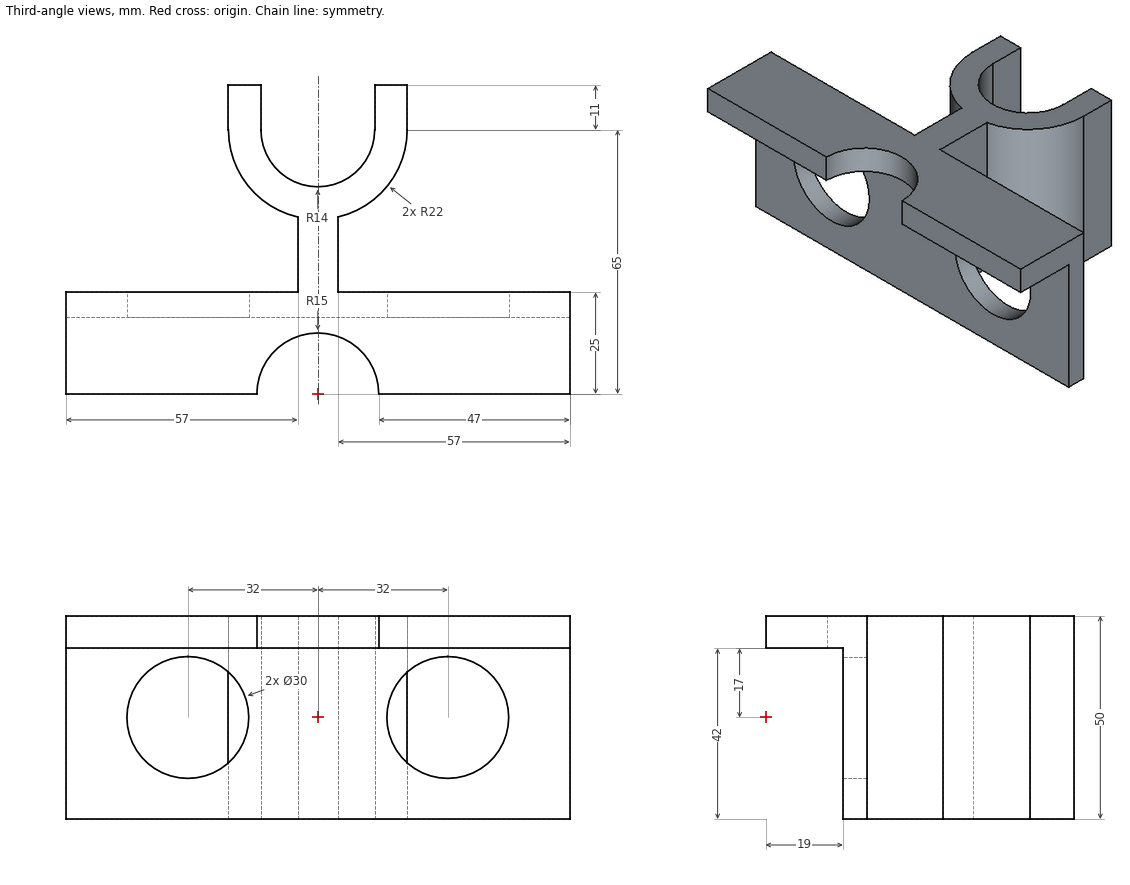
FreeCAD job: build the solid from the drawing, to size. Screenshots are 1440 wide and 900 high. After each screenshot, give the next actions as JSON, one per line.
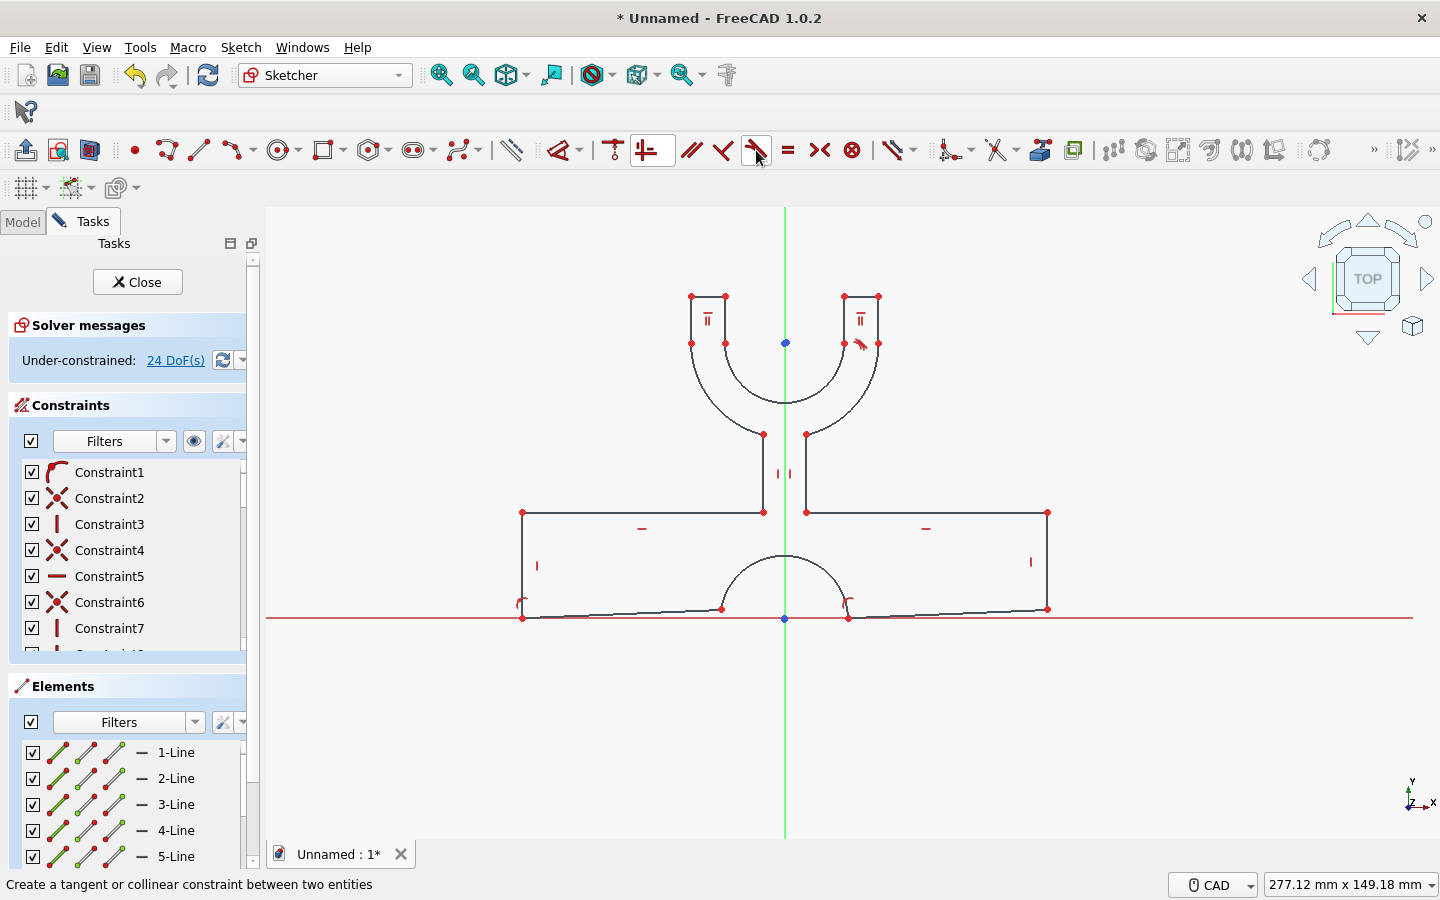
{"action": "left_click", "coordinate": [725, 330]}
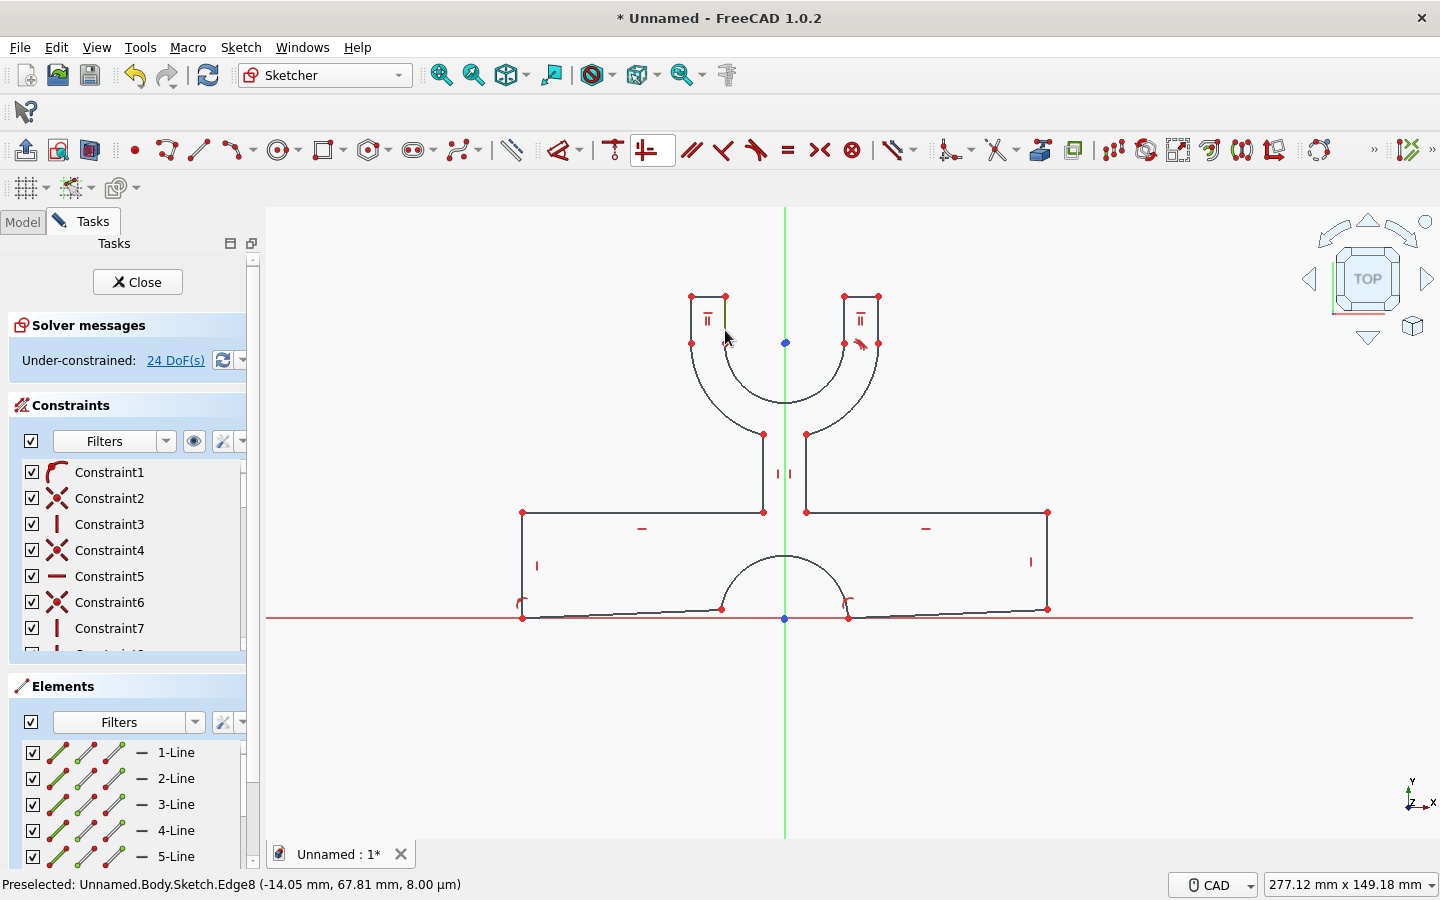
{"action": "left_click", "coordinate": [750, 392]}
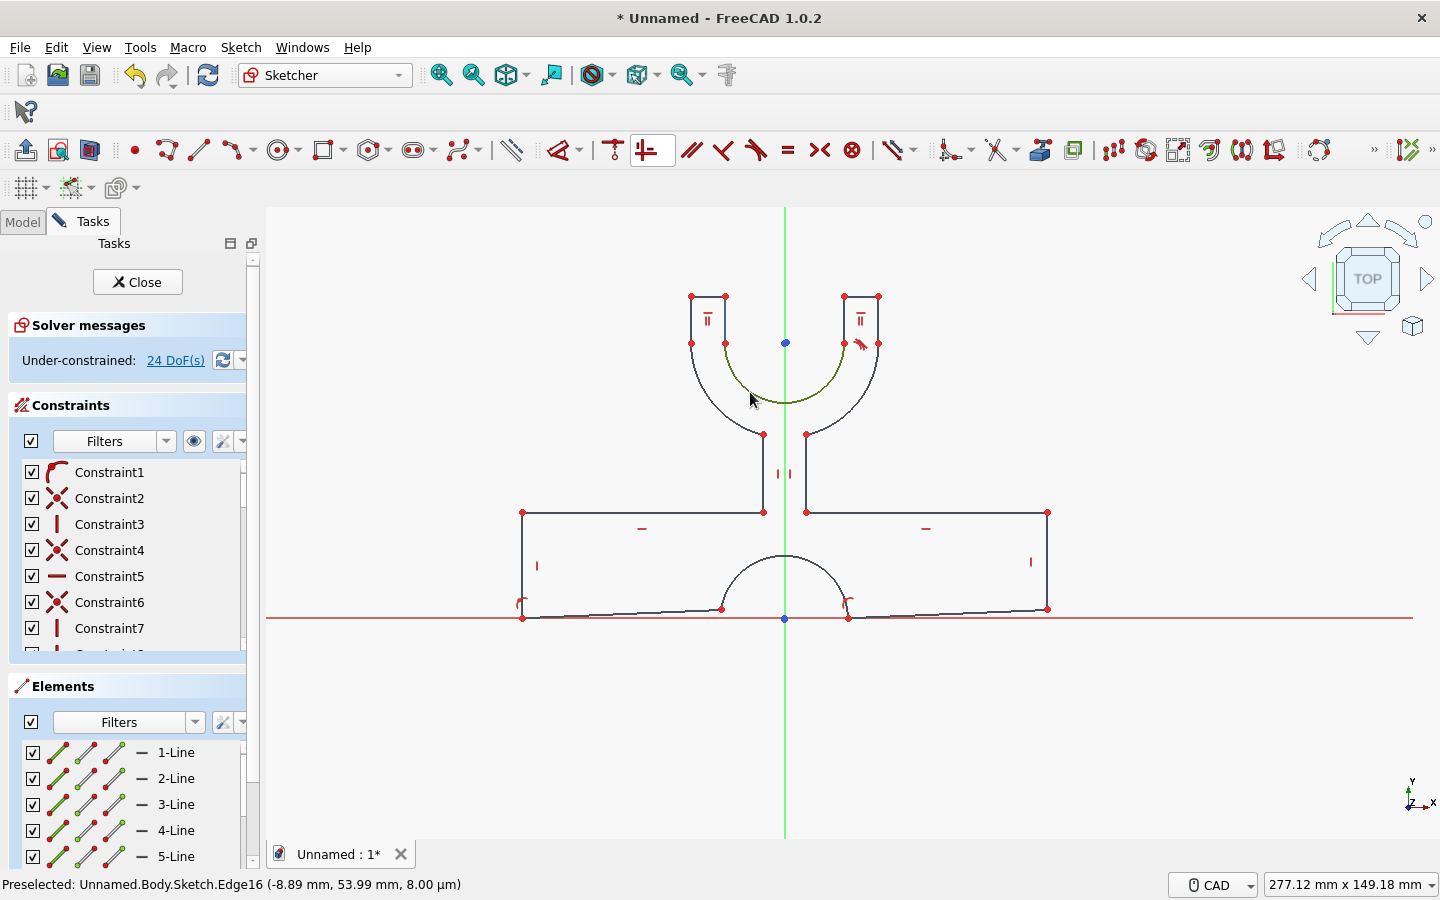
{"action": "left_click", "coordinate": [756, 150]}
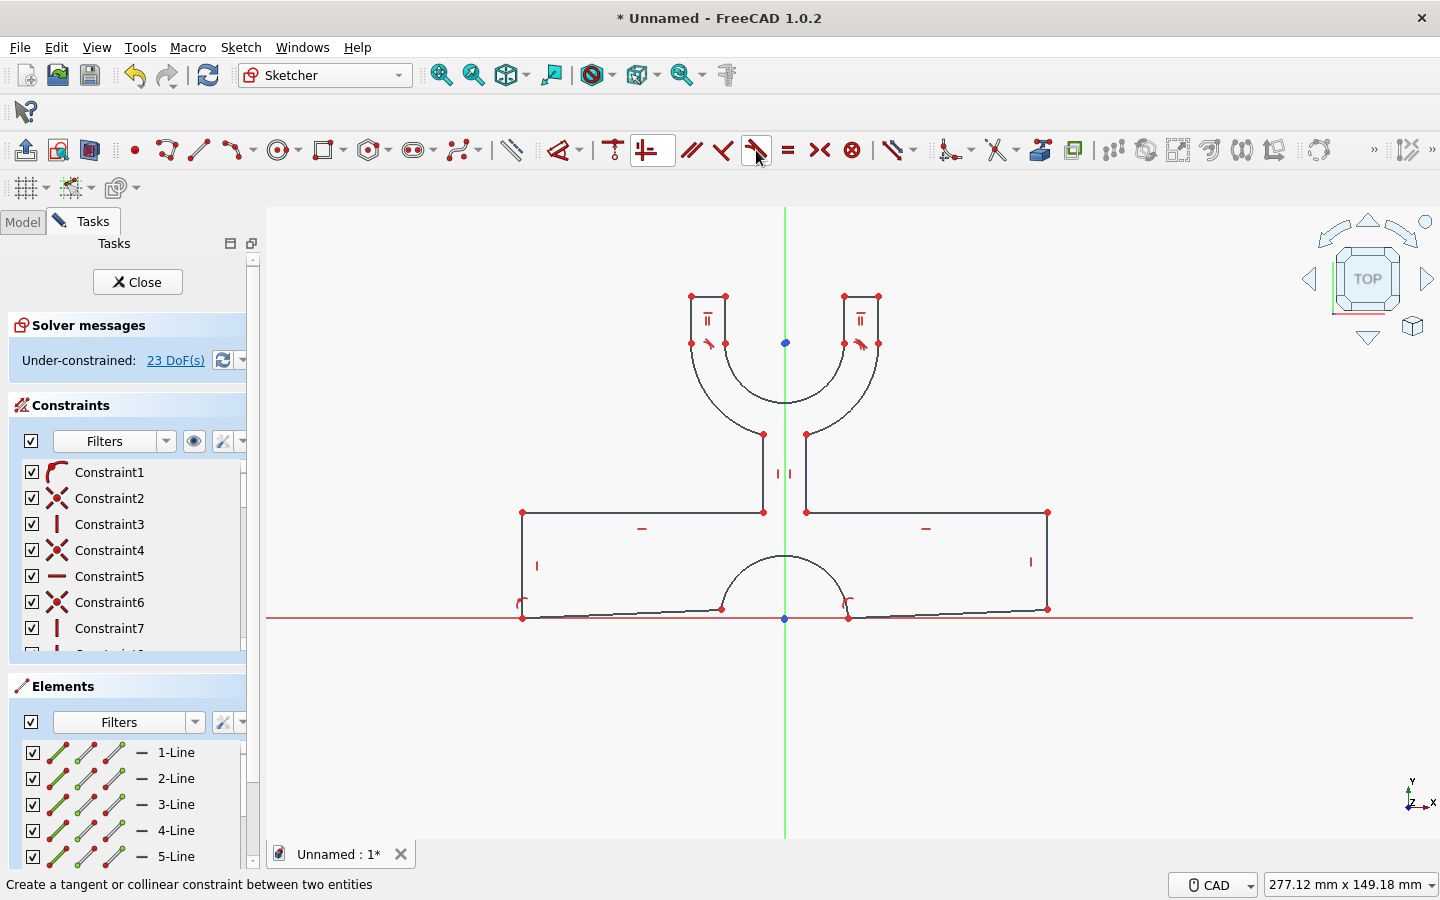
{"action": "left_click", "coordinate": [691, 311]}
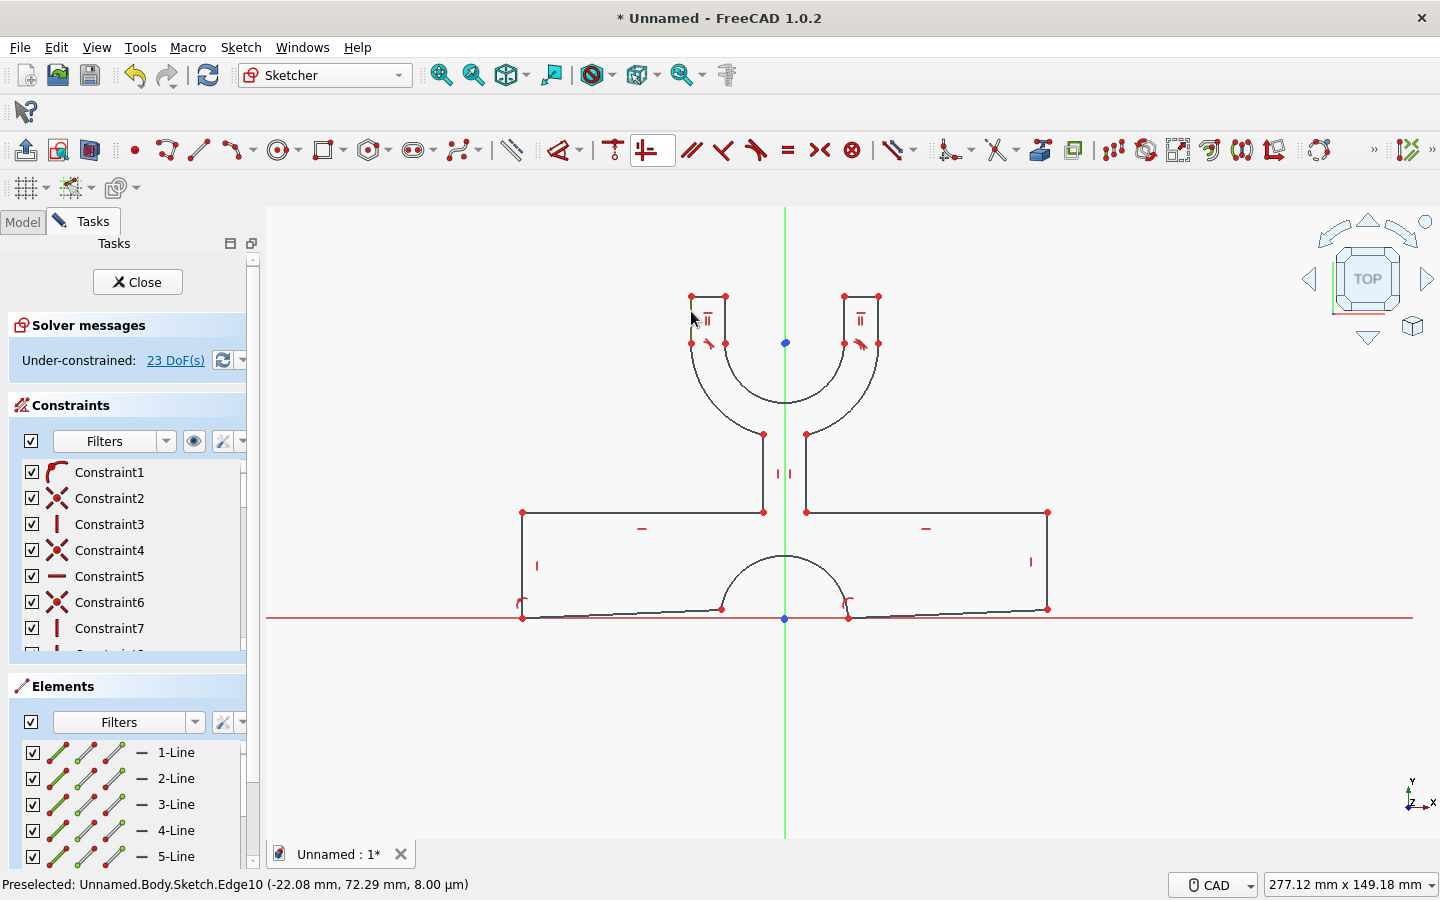
{"action": "left_click", "coordinate": [699, 380]}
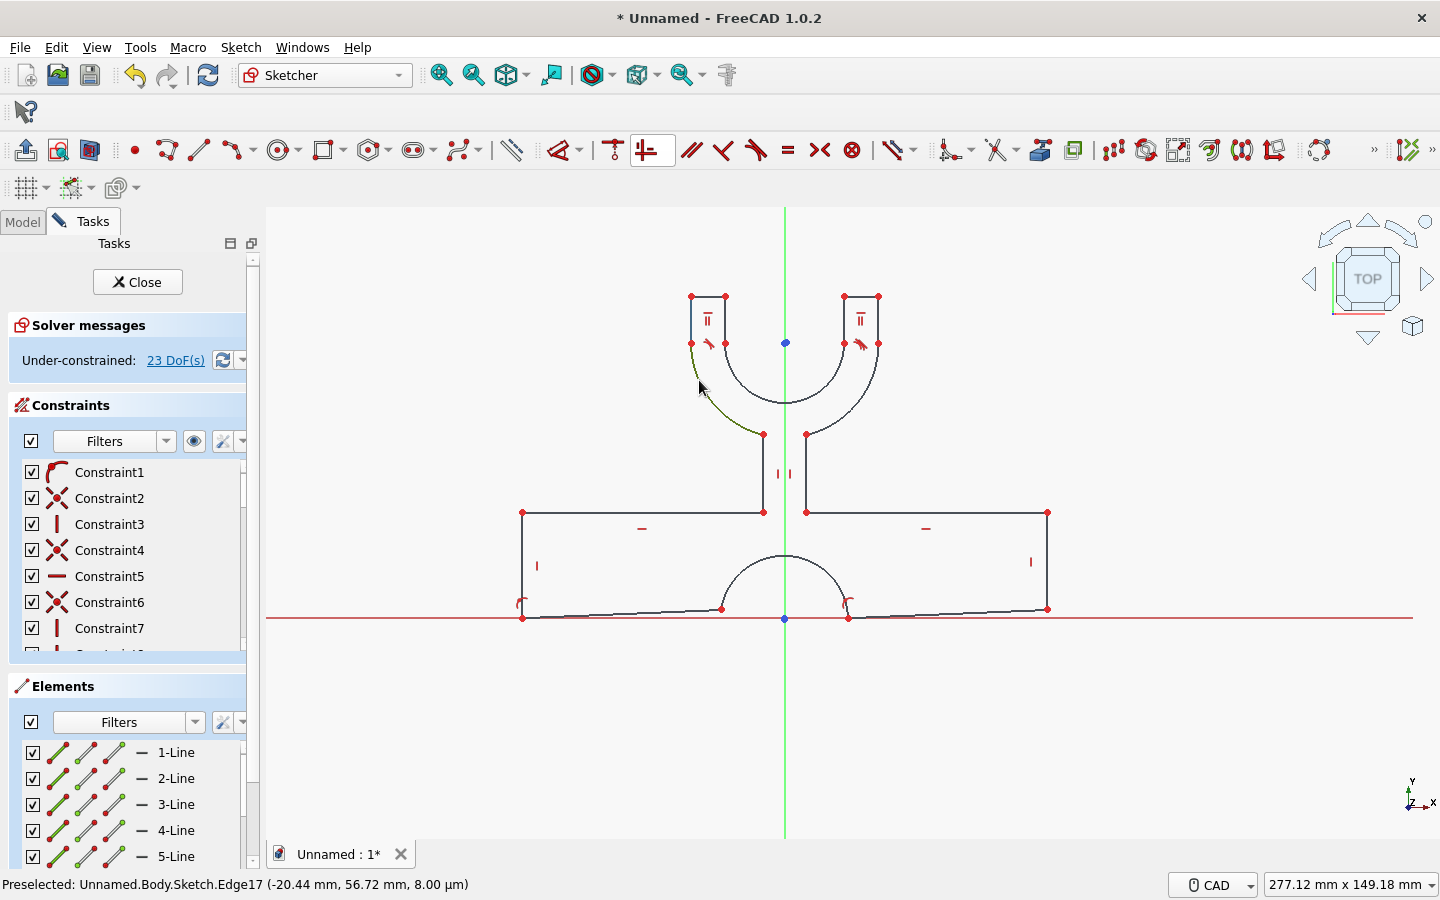
{"action": "left_click", "coordinate": [756, 150]}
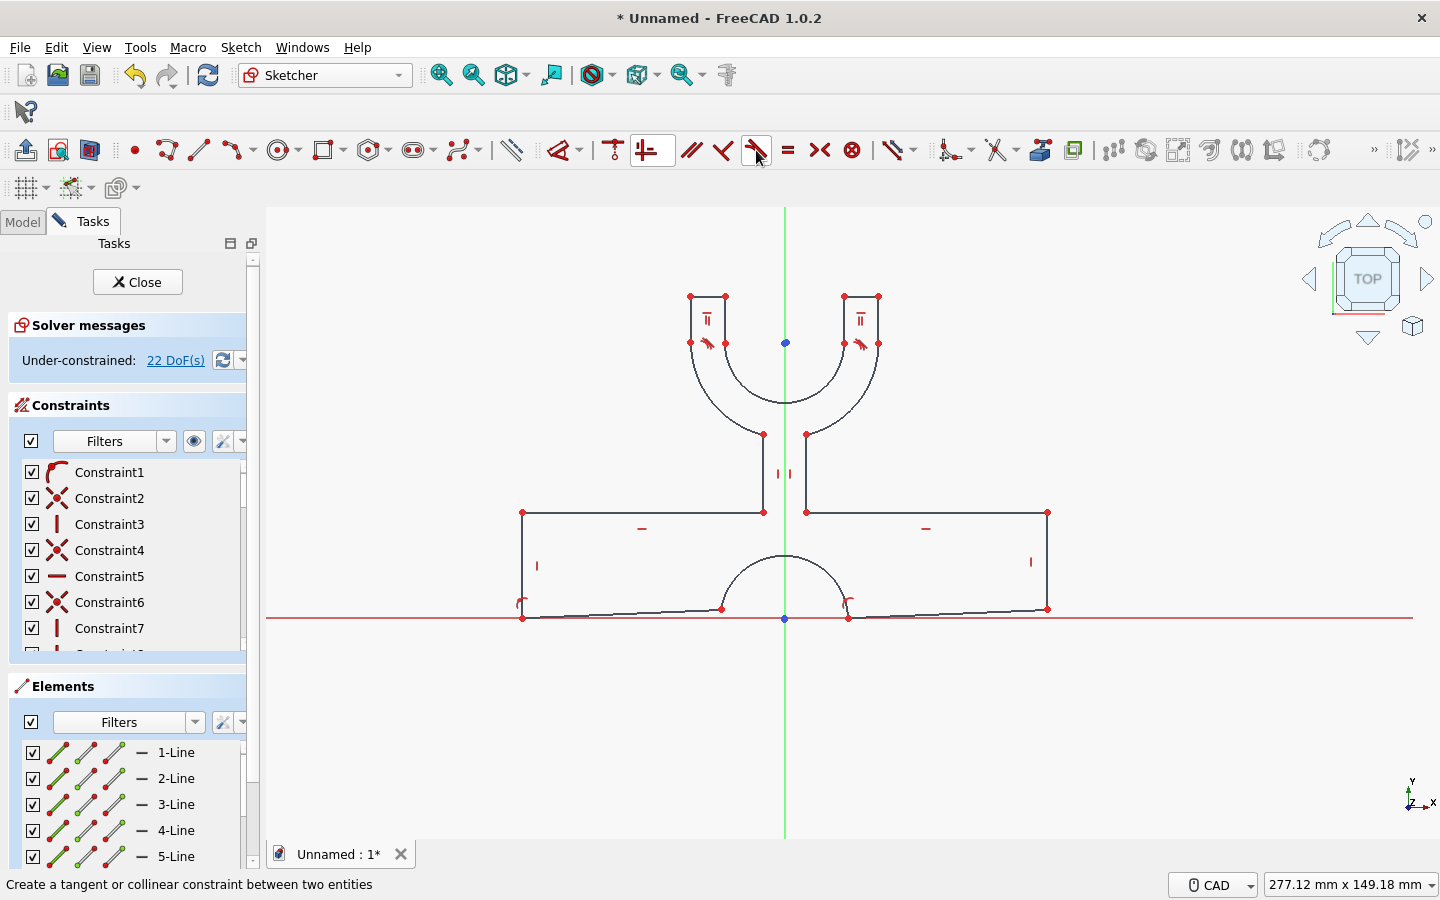
{"action": "left_click", "coordinate": [908, 616]}